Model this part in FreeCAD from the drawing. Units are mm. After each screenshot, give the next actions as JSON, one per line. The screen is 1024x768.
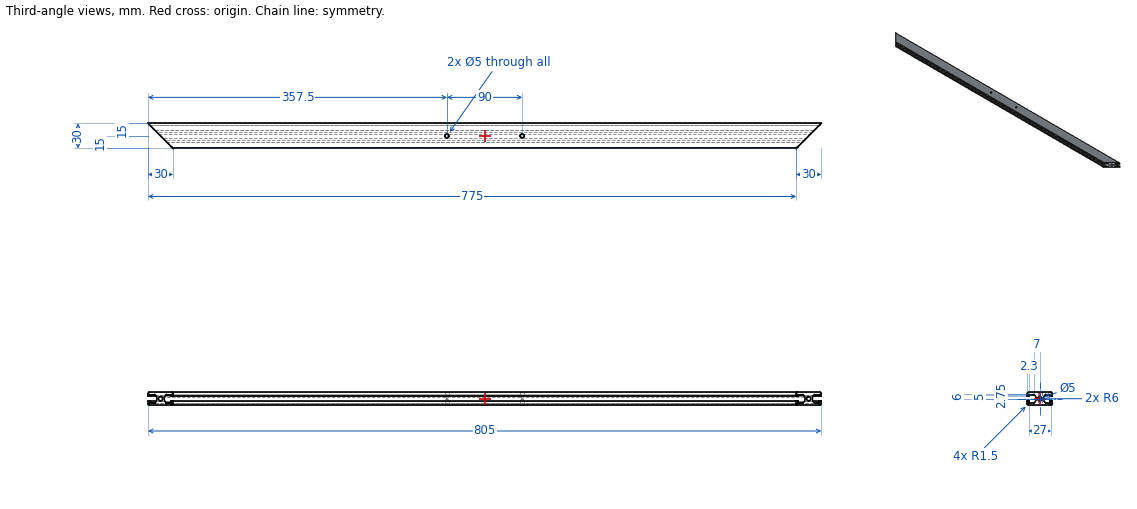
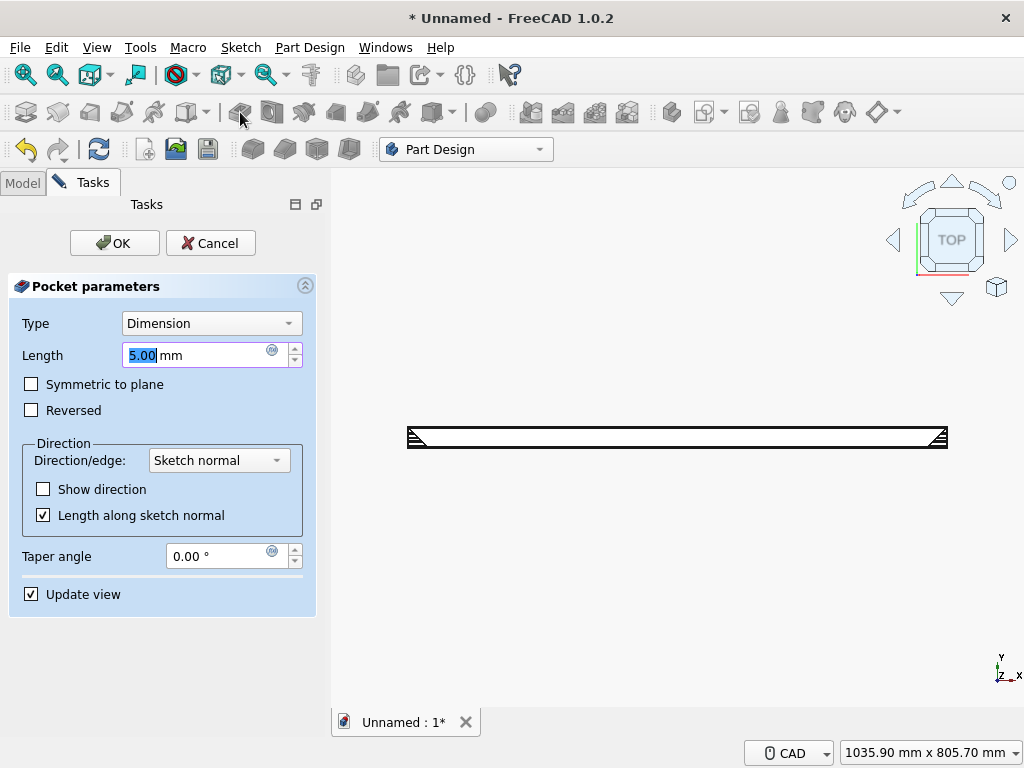
{"action": "left_click", "coordinate": [212, 324]}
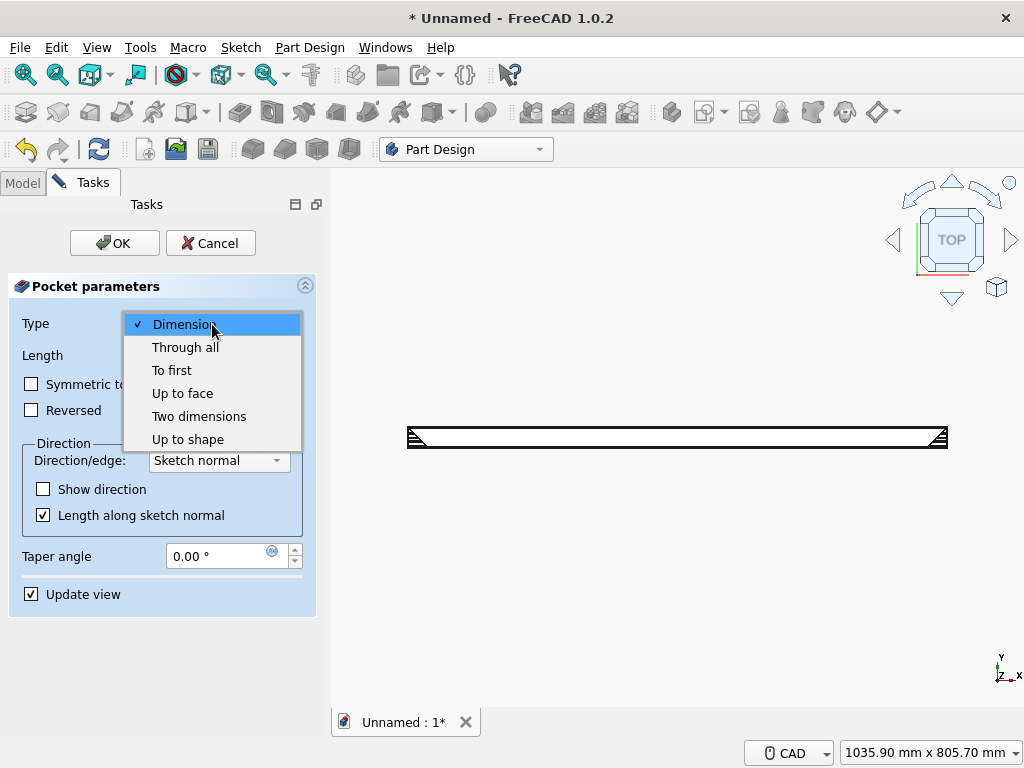
{"action": "left_click", "coordinate": [212, 348]}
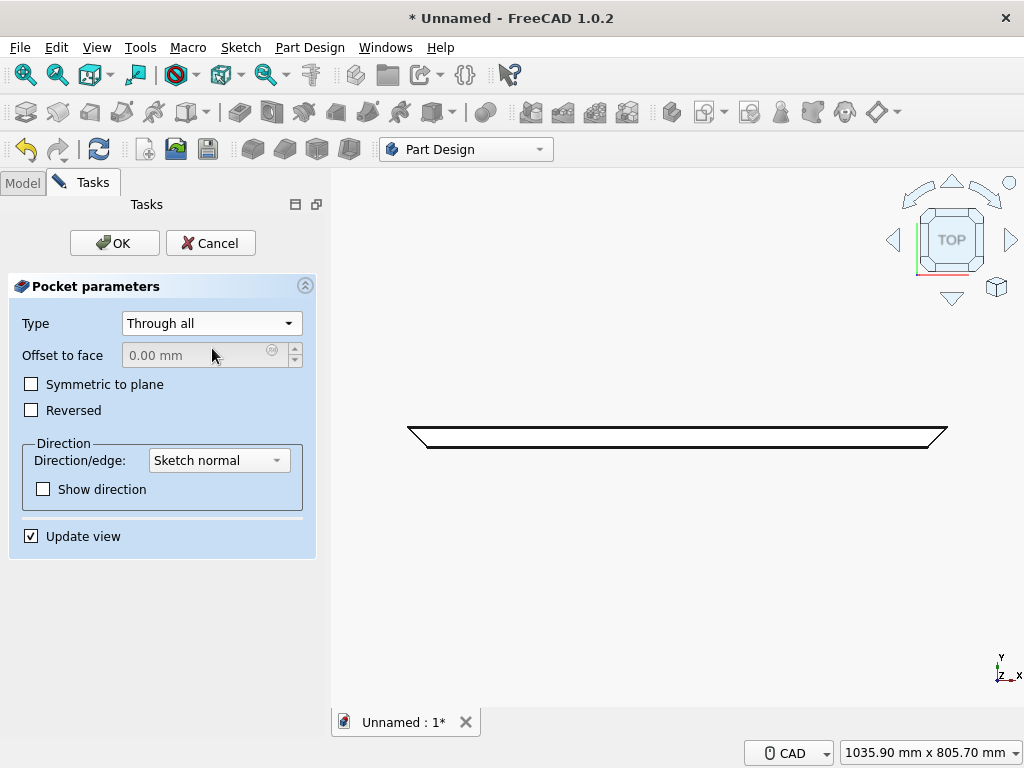
{"action": "left_click", "coordinate": [115, 243]}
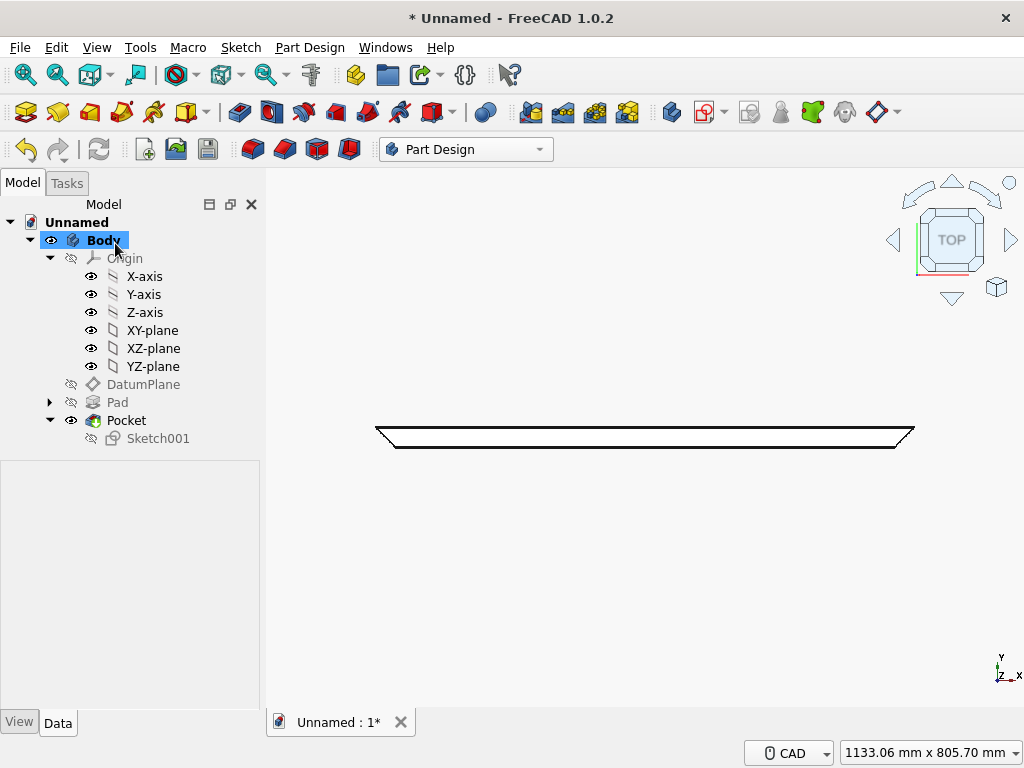
{"action": "left_click", "coordinate": [645, 436]}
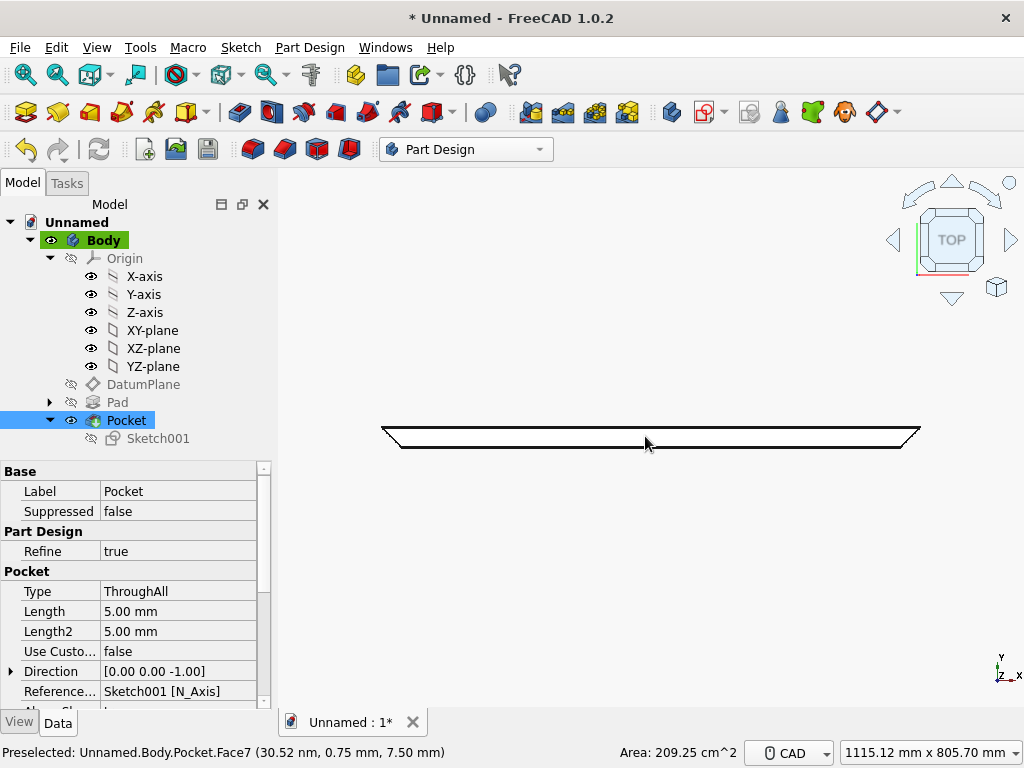
{"action": "left_click", "coordinate": [704, 112]}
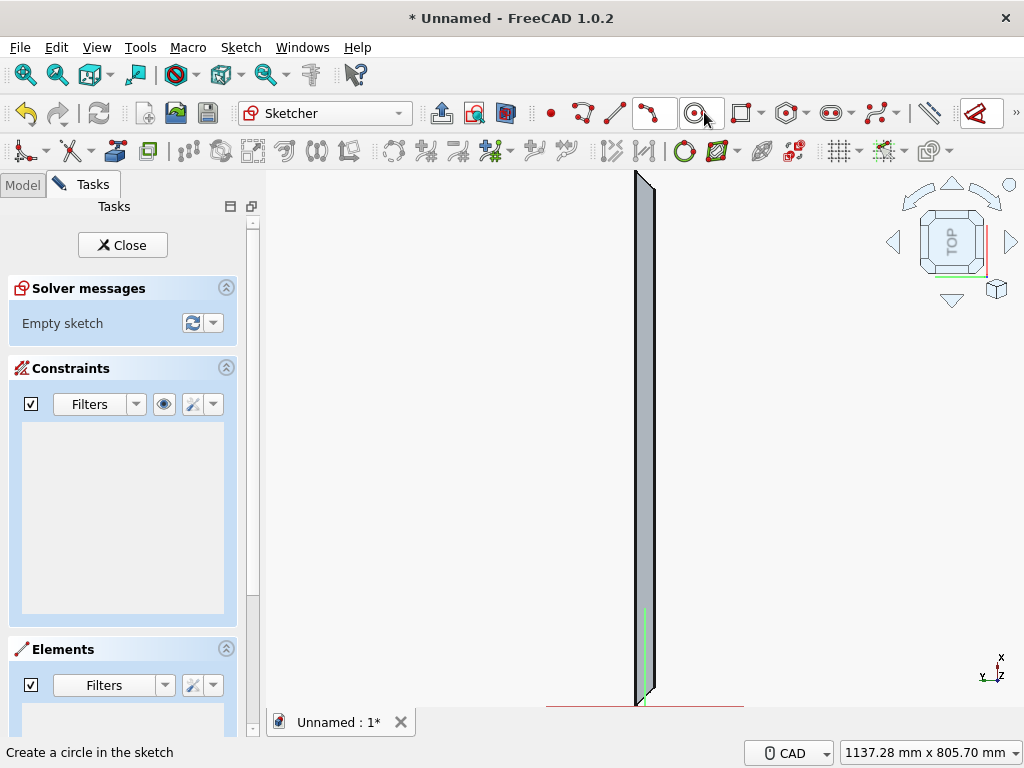
{"action": "scroll", "coordinate": [662, 439], "scroll_direction": "up", "scroll_amount": 8}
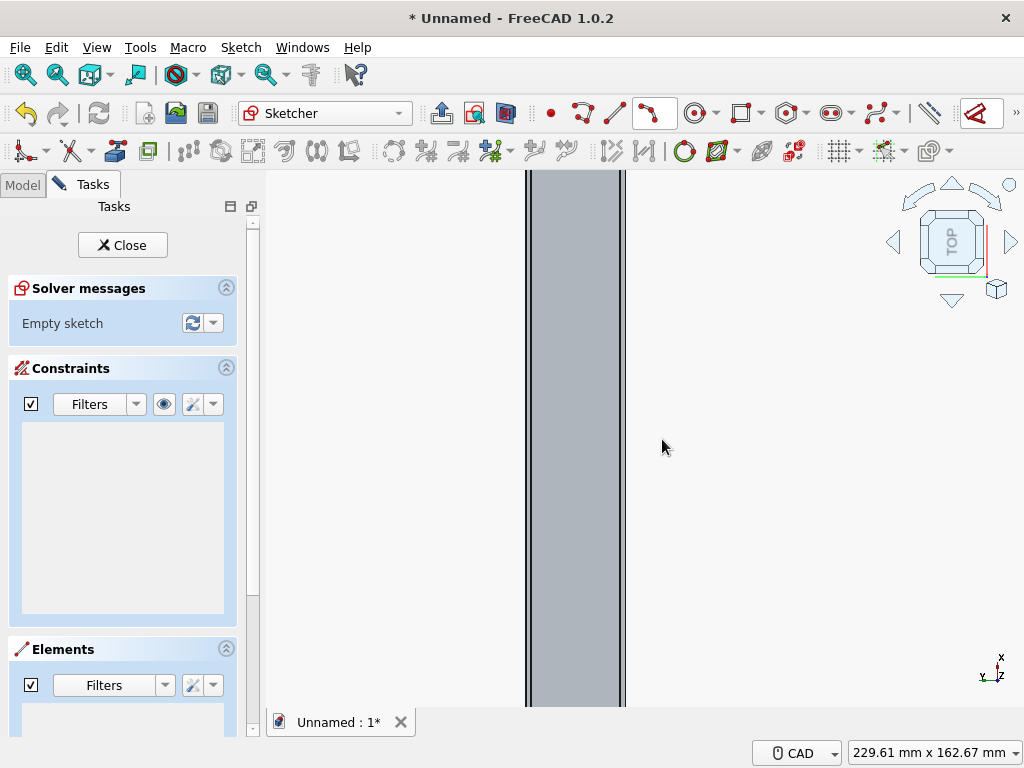
{"action": "left_click", "coordinate": [696, 114]}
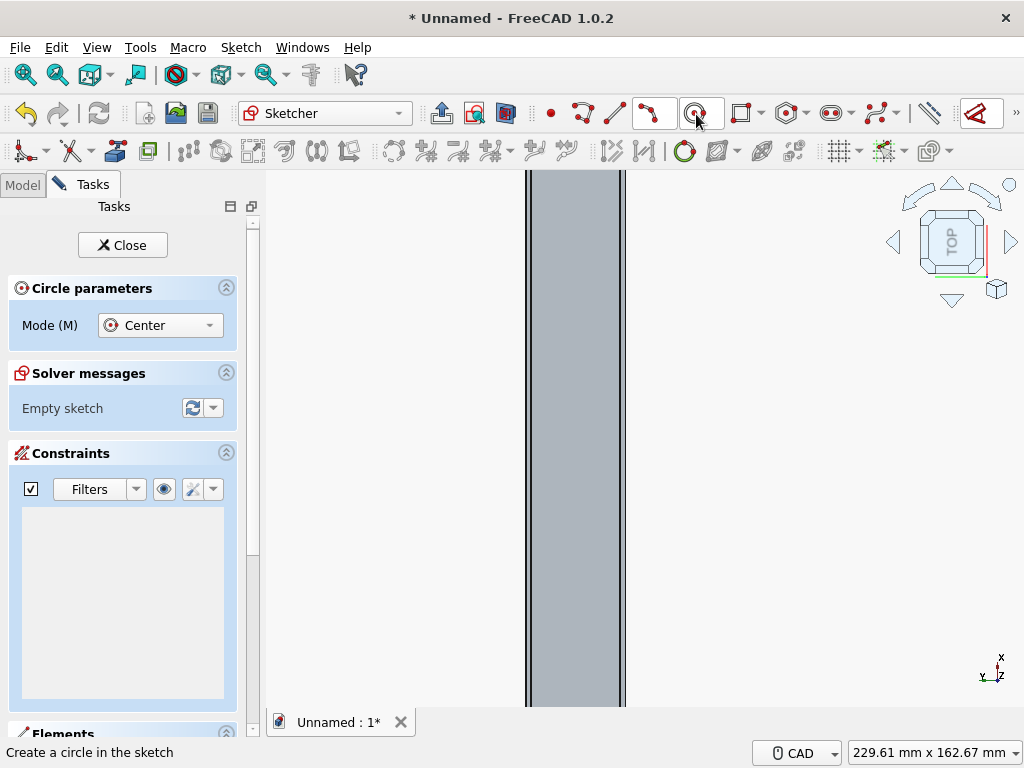
{"action": "scroll", "coordinate": [576, 583], "scroll_direction": "up", "scroll_amount": 6}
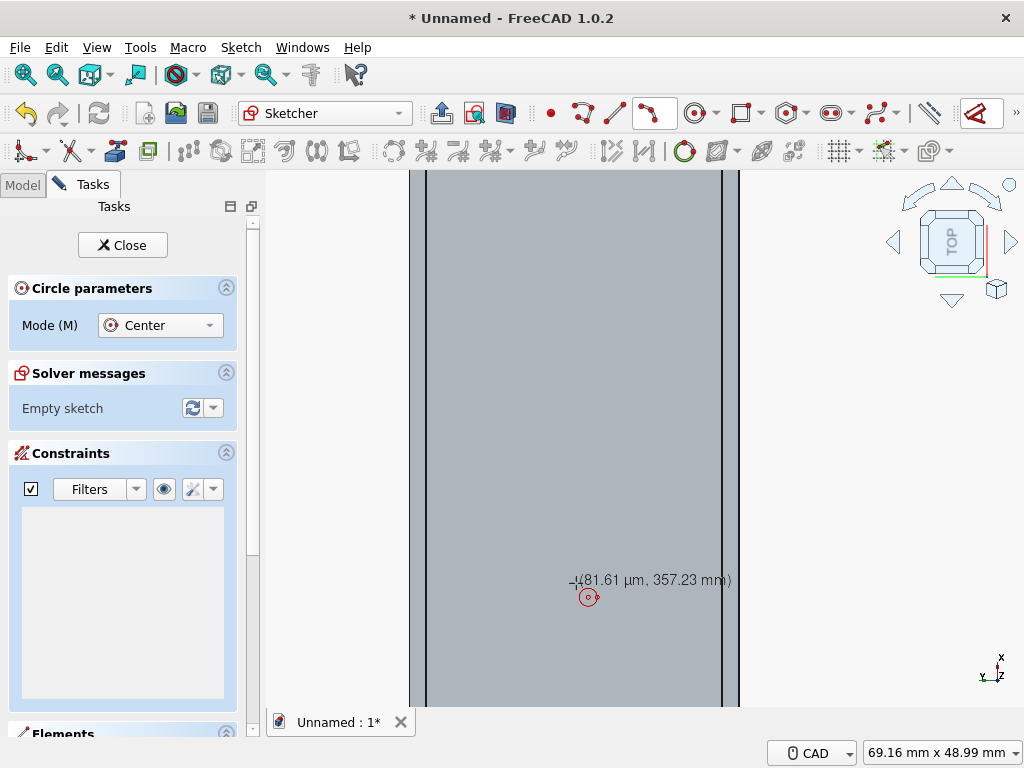
{"action": "left_click", "coordinate": [574, 582]}
{"action": "mouse_move", "coordinate": [594, 562]}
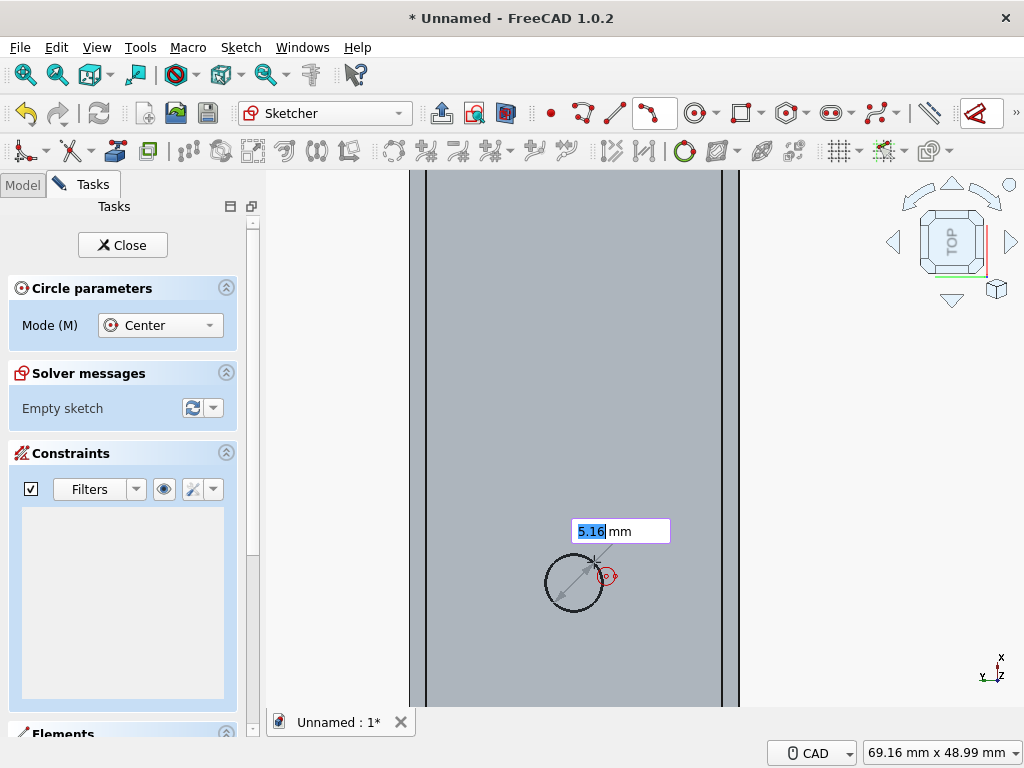
{"action": "type", "text": "5"}
{"action": "key", "text": "Return"}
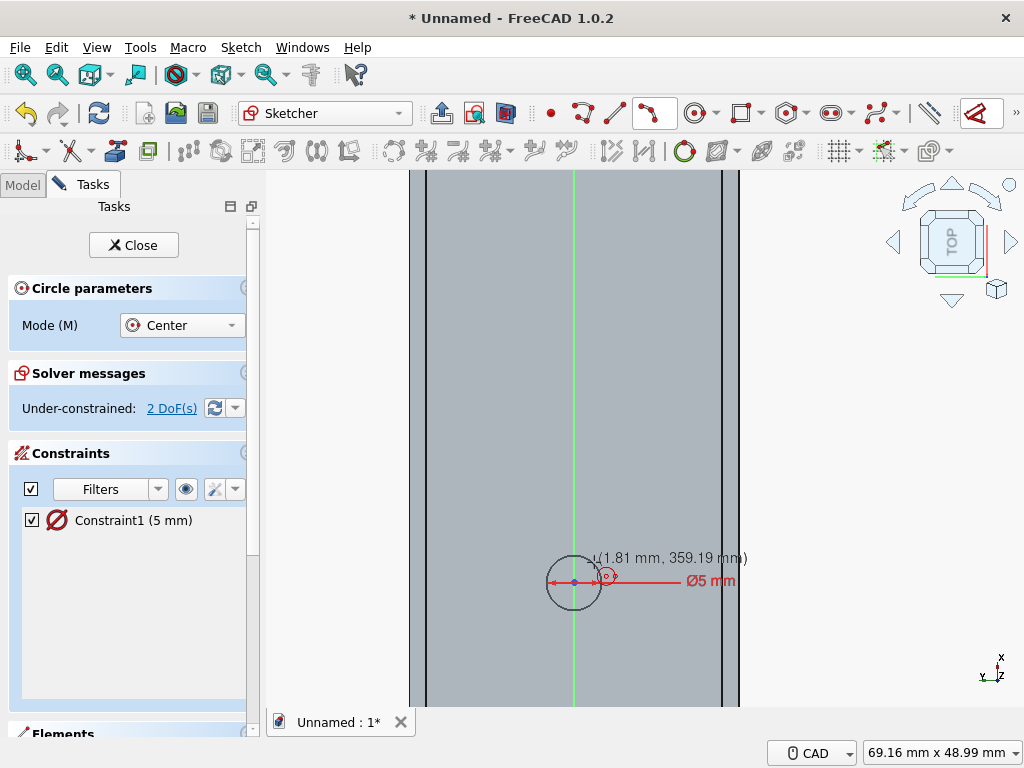
{"action": "scroll", "coordinate": [578, 589], "scroll_direction": "down", "scroll_amount": 6}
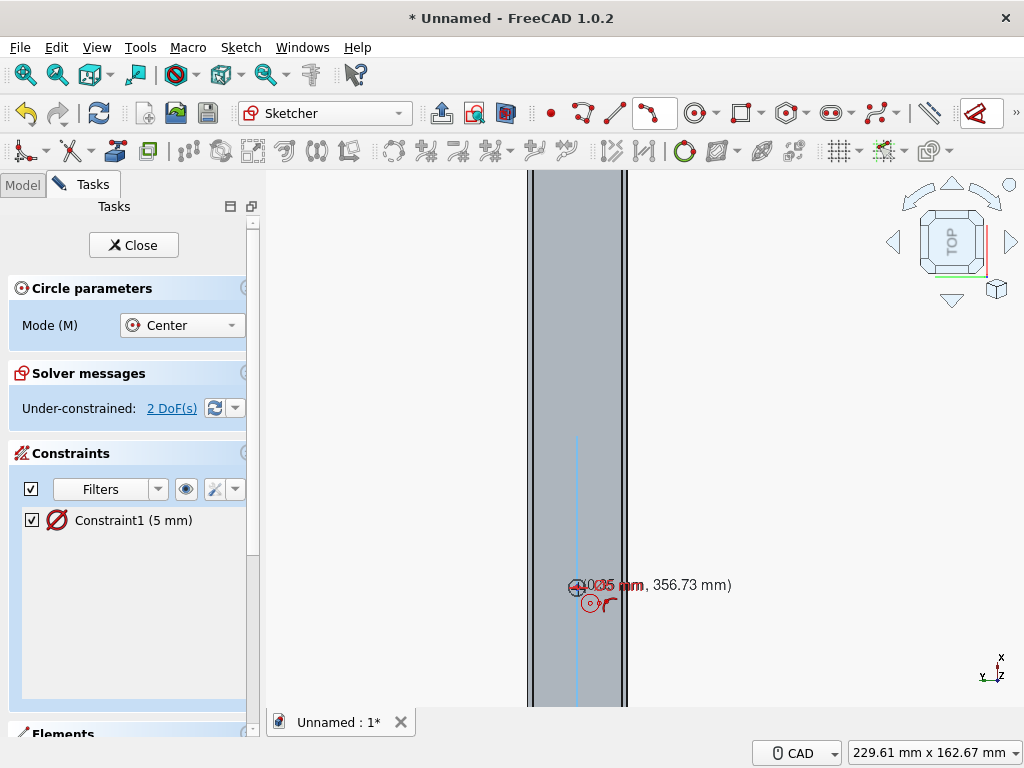
{"action": "scroll", "coordinate": [577, 290], "scroll_direction": "up", "scroll_amount": 6}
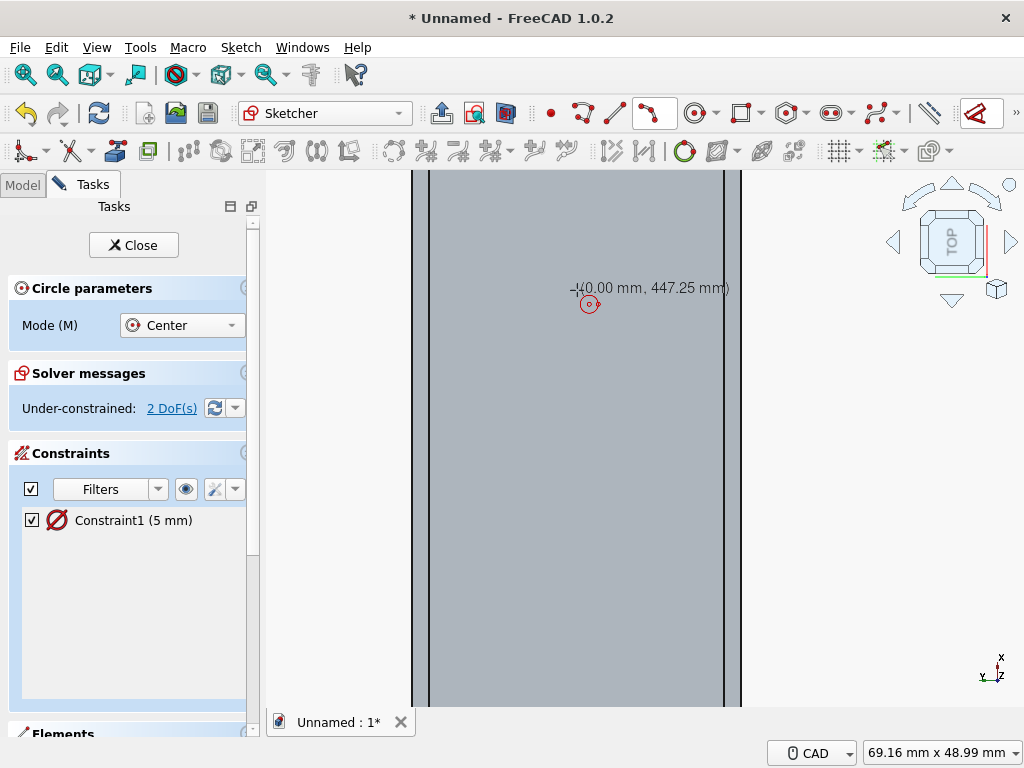
{"action": "left_click", "coordinate": [576, 290]}
{"action": "mouse_move", "coordinate": [596, 271]}